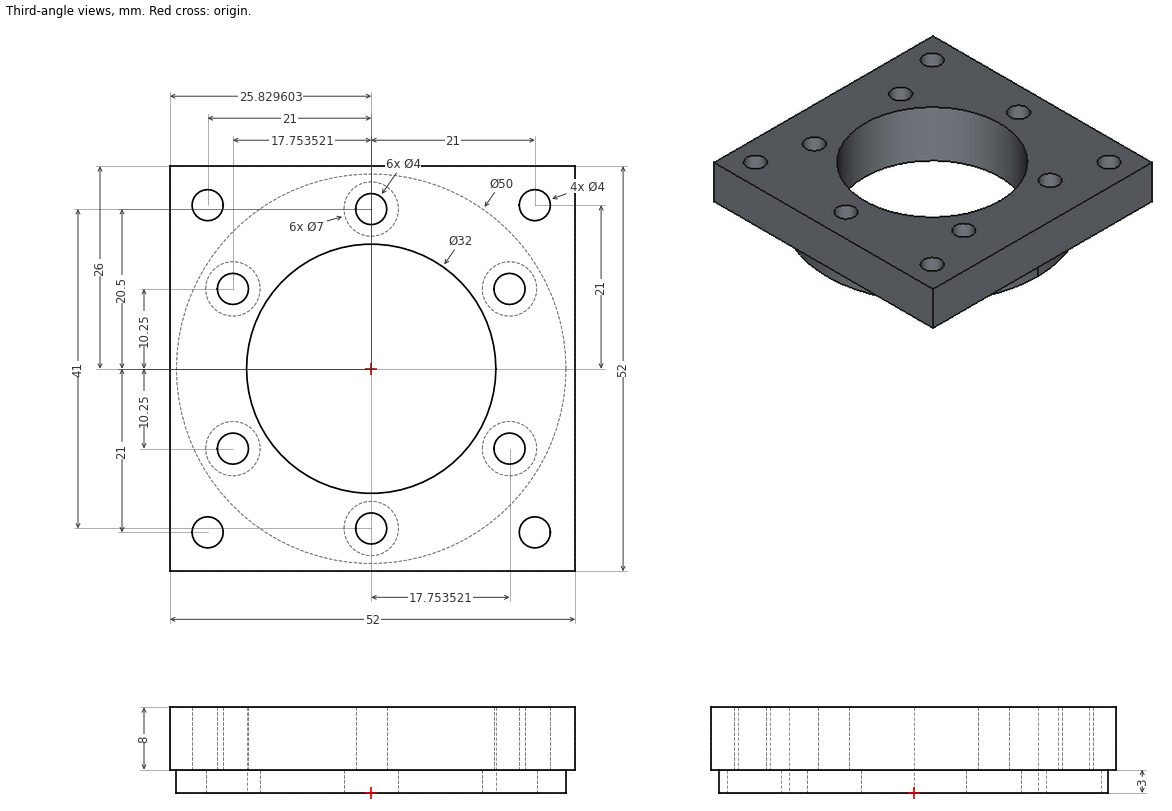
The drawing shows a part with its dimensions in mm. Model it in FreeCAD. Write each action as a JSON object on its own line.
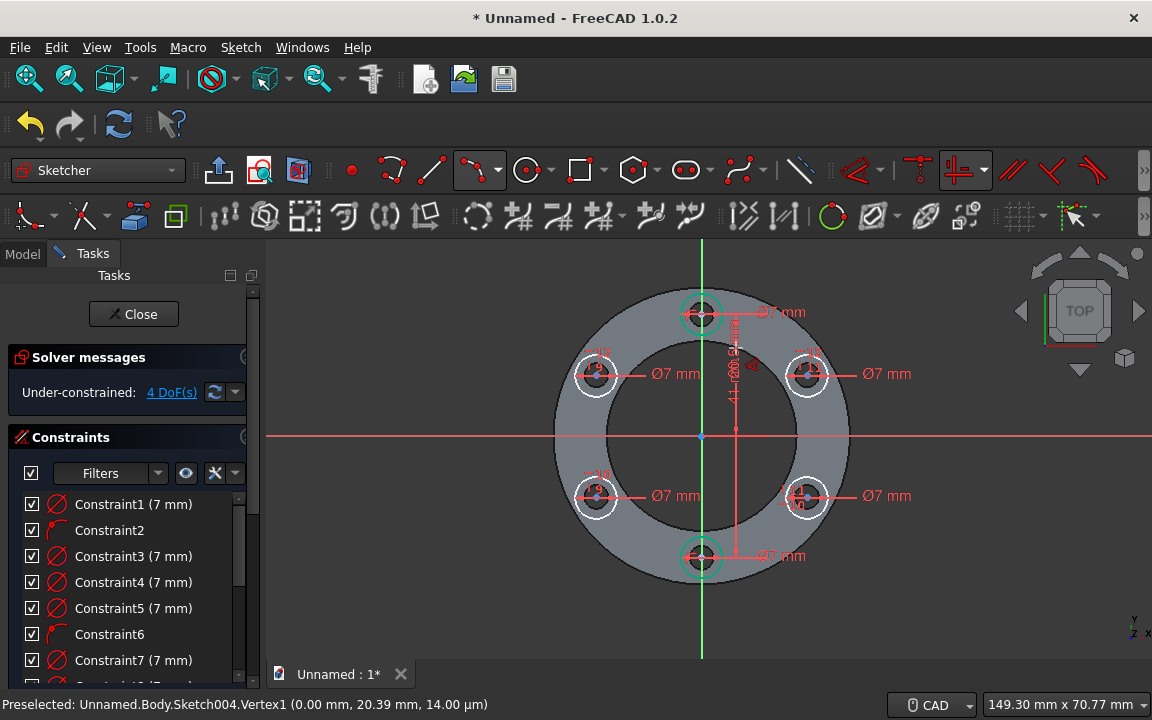
{"action": "left_click", "coordinate": [596, 376]}
{"action": "left_click", "coordinate": [562, 406]}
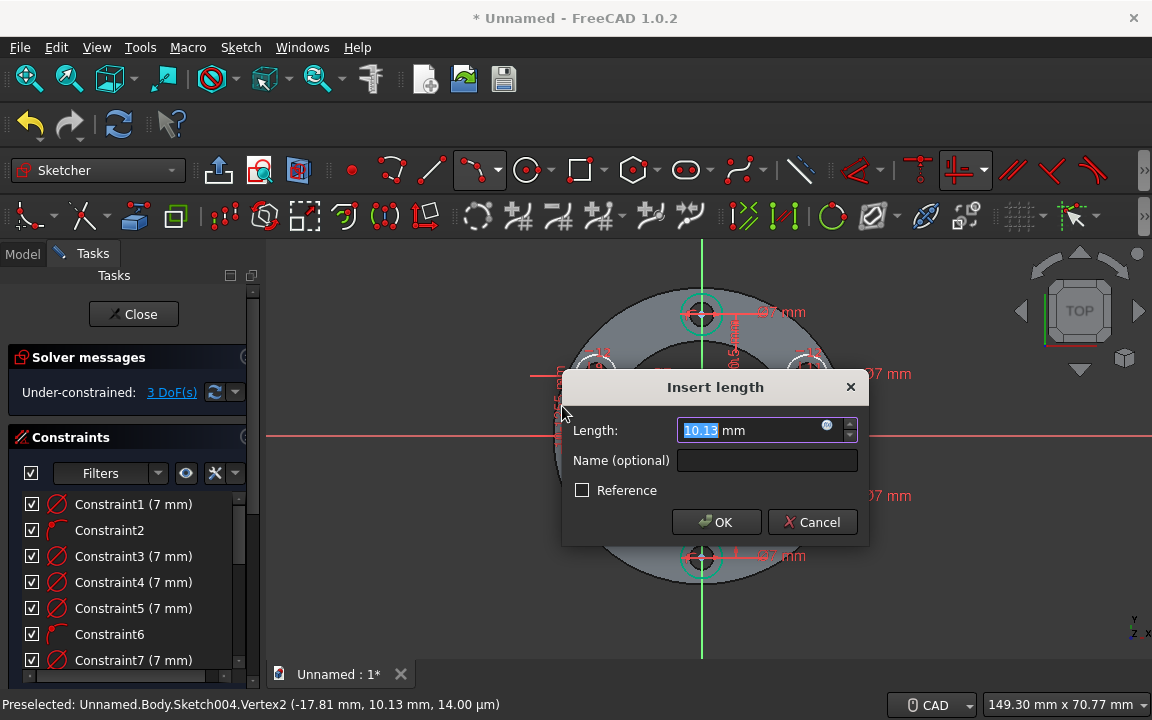
{"action": "type", "text": "10.25"}
{"action": "key", "text": "Return"}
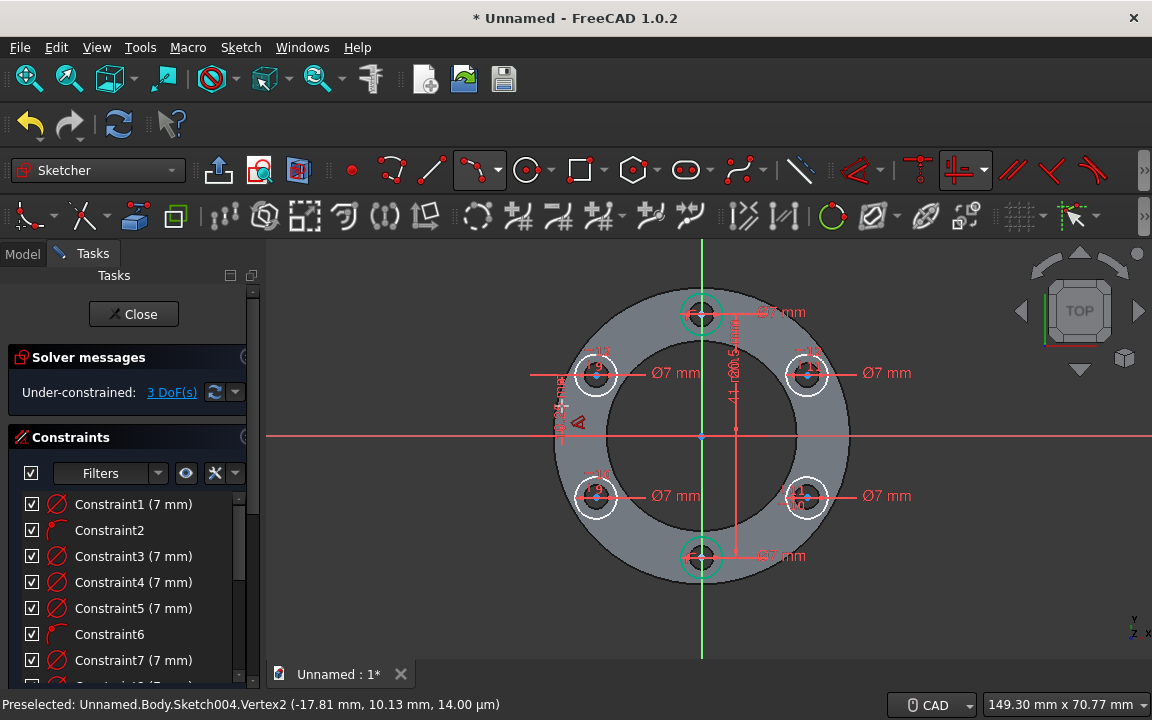
{"action": "left_click", "coordinate": [596, 498]}
{"action": "left_click", "coordinate": [562, 467]}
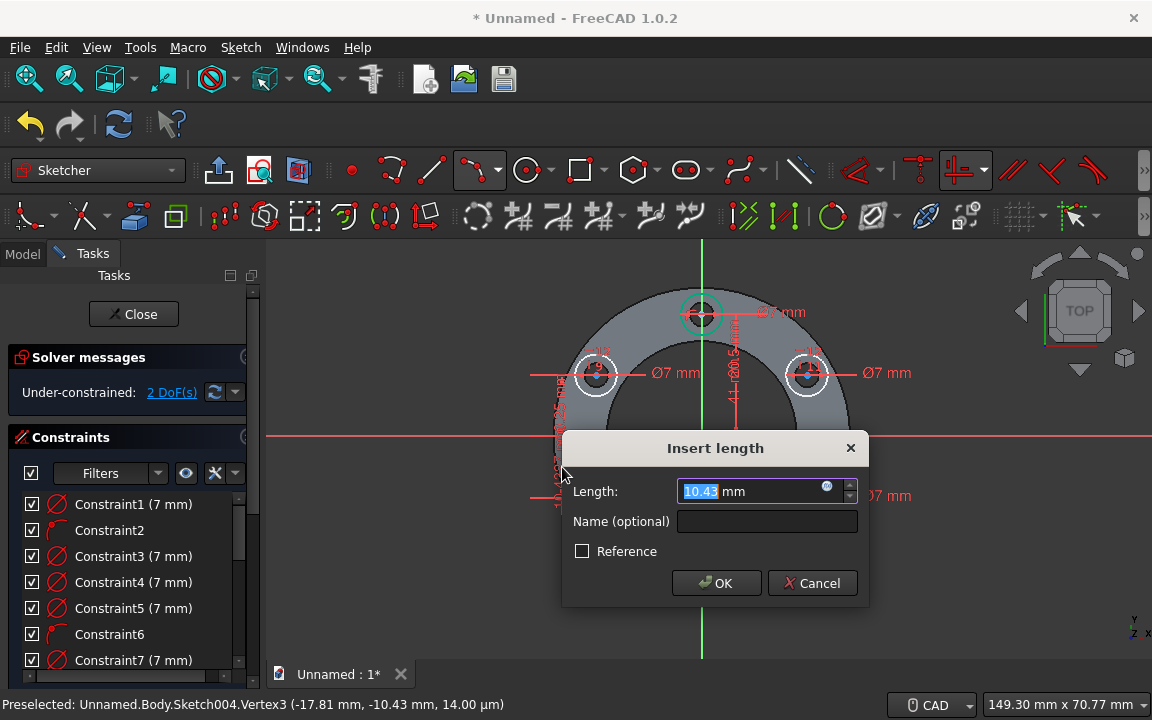
{"action": "type", "text": "10.25"}
{"action": "key", "text": "Return"}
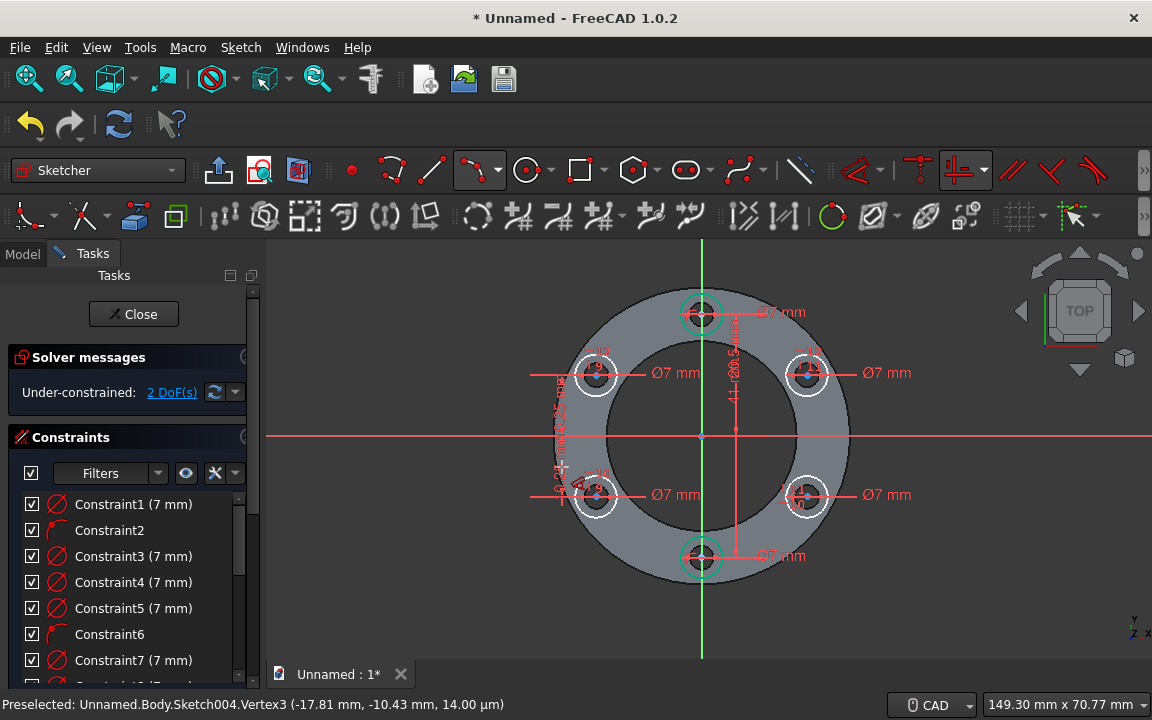
{"action": "left_click", "coordinate": [596, 375]}
{"action": "left_click", "coordinate": [649, 341]}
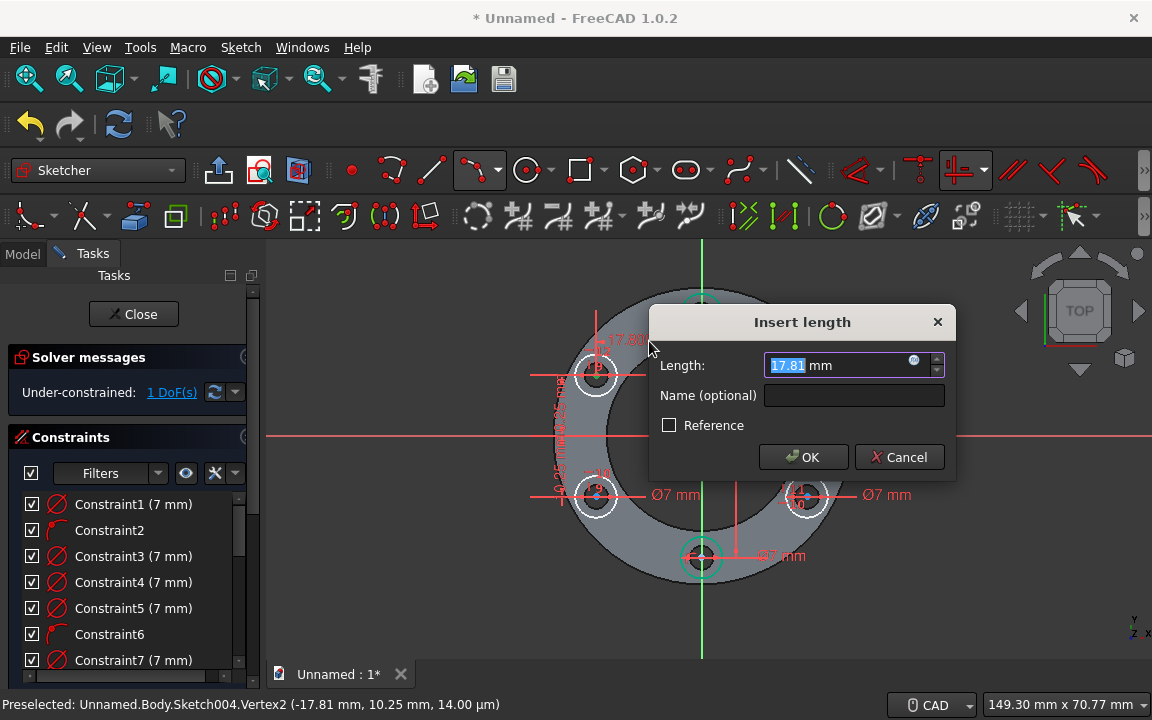
{"action": "type", "text": "17.753521"}
{"action": "key", "text": "Return"}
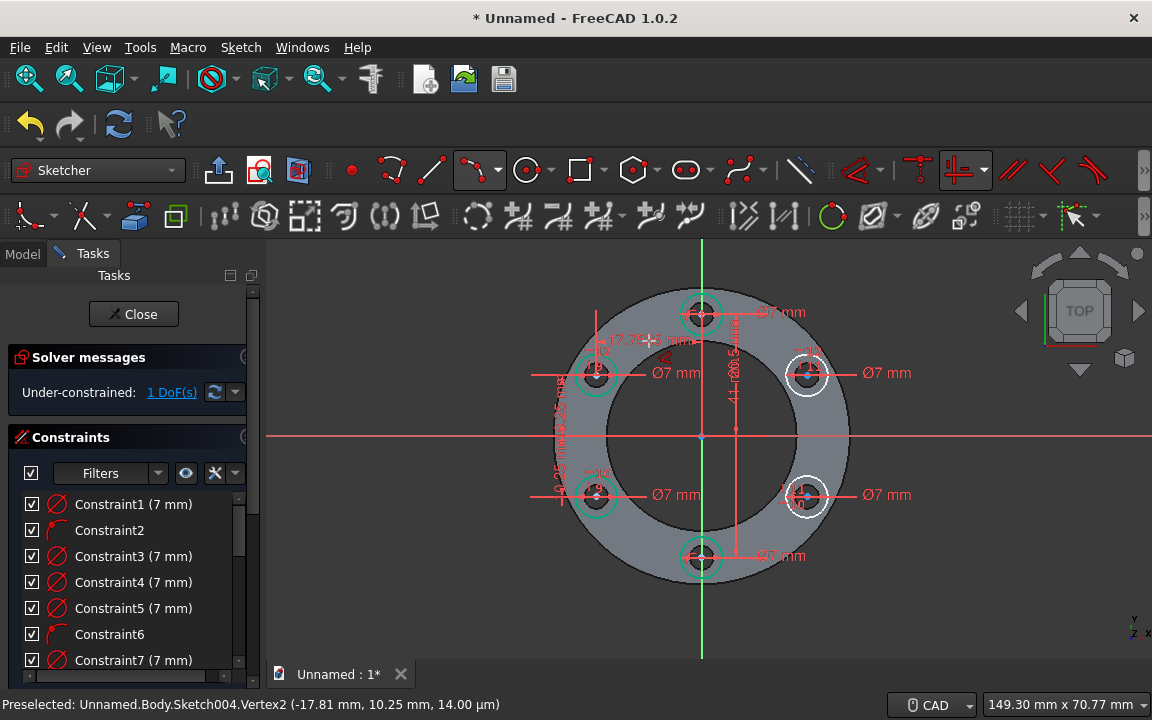
{"action": "left_click", "coordinate": [807, 497]}
{"action": "left_click", "coordinate": [754, 531]}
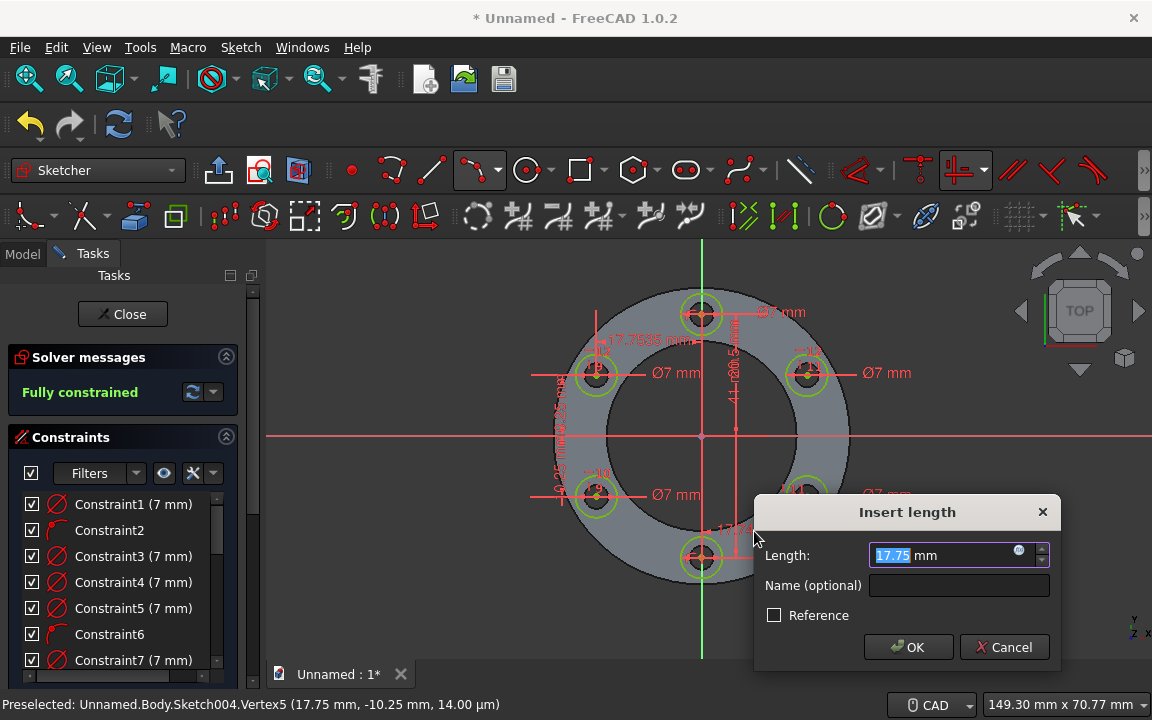
{"action": "type", "text": "17.753521"}
{"action": "key", "text": "Return"}
{"action": "key", "text": "Escape"}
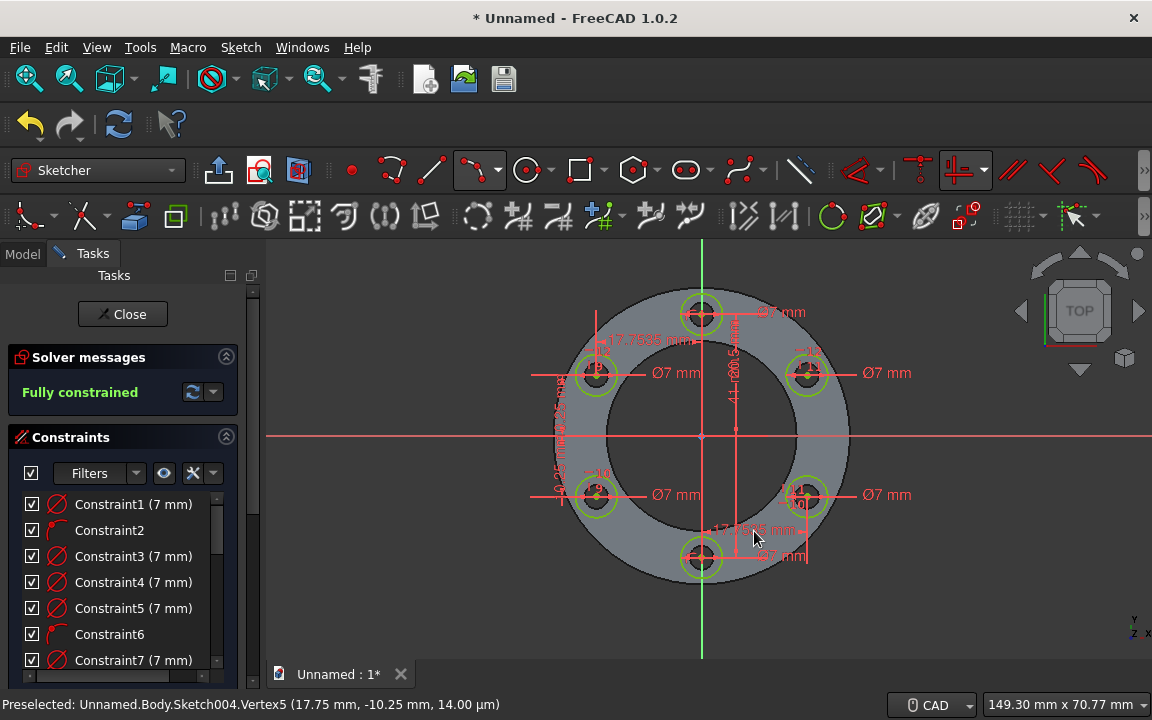
{"action": "left_click", "coordinate": [123, 314]}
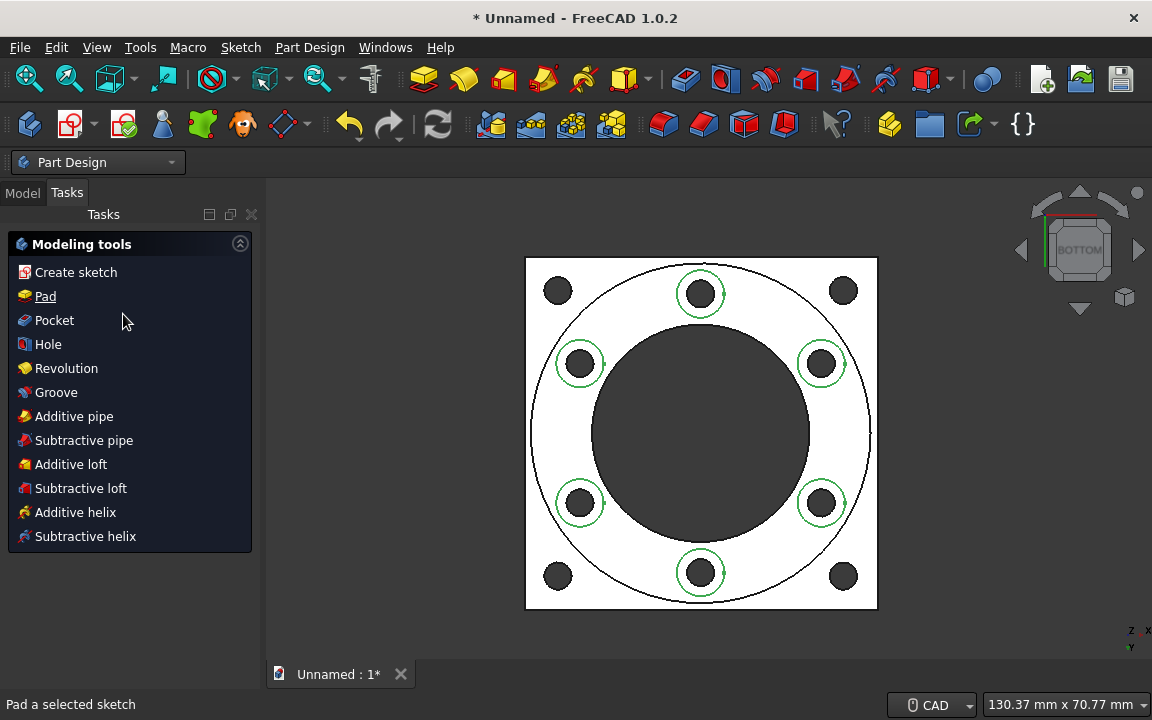
{"action": "left_click", "coordinate": [686, 80]}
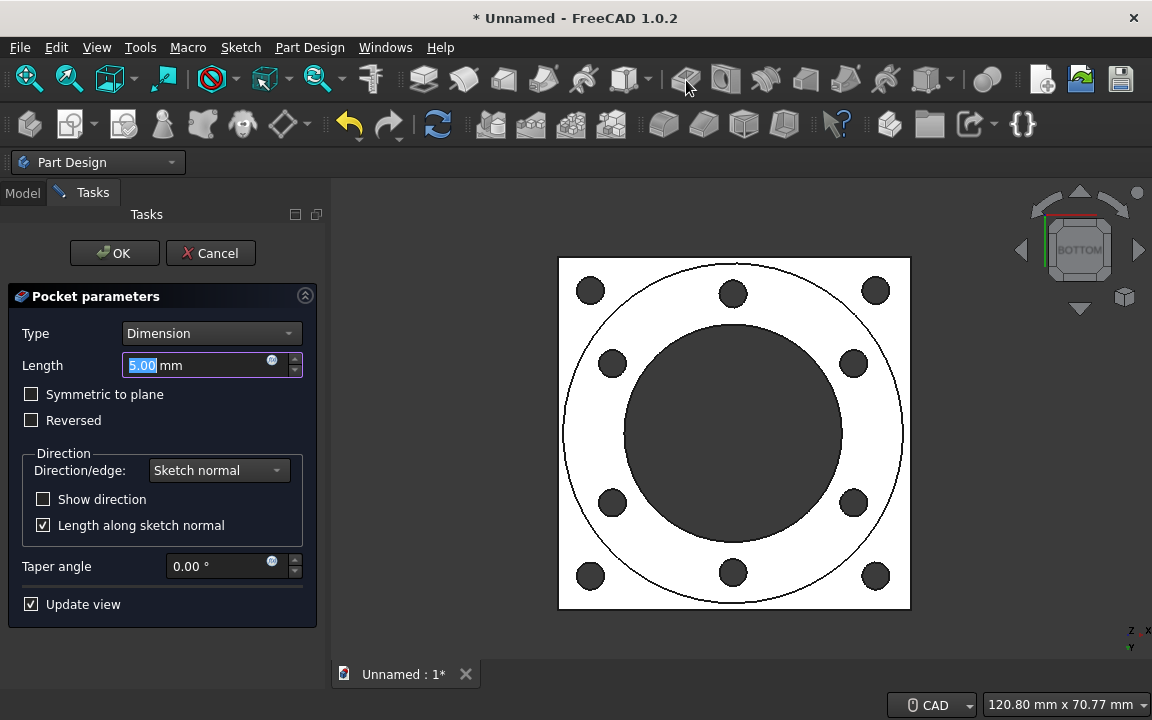
{"action": "type", "text": "3"}
{"action": "key", "text": "Tab"}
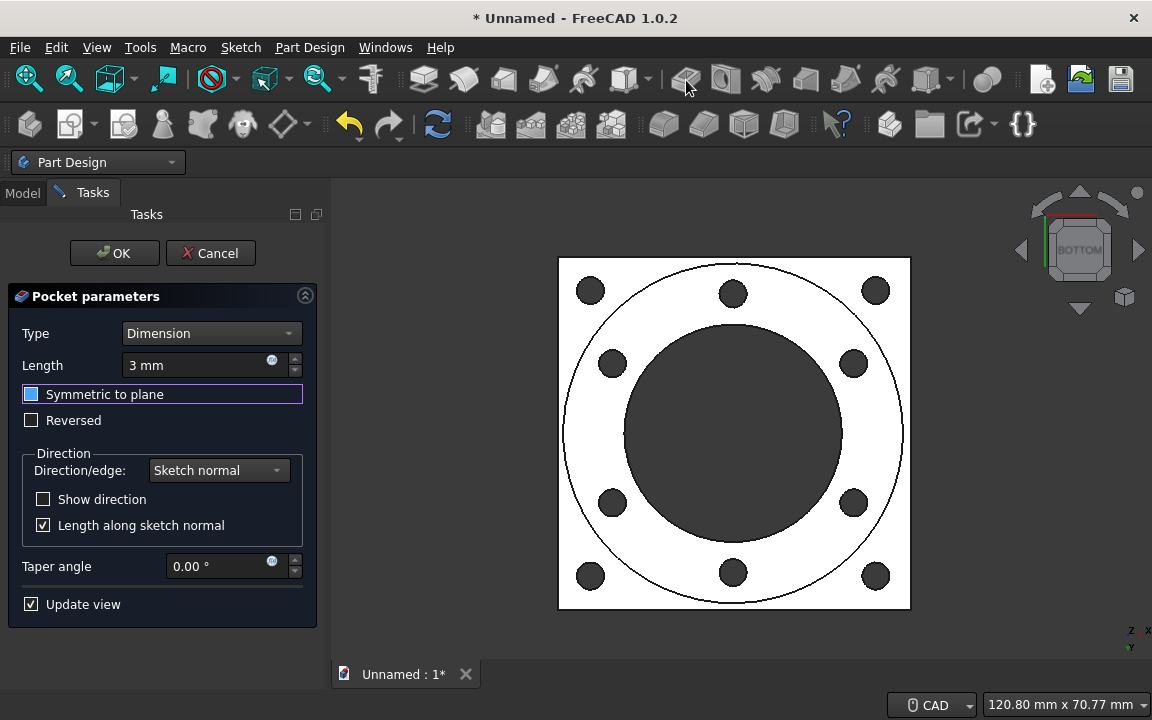
{"action": "left_click", "coordinate": [30, 420]}